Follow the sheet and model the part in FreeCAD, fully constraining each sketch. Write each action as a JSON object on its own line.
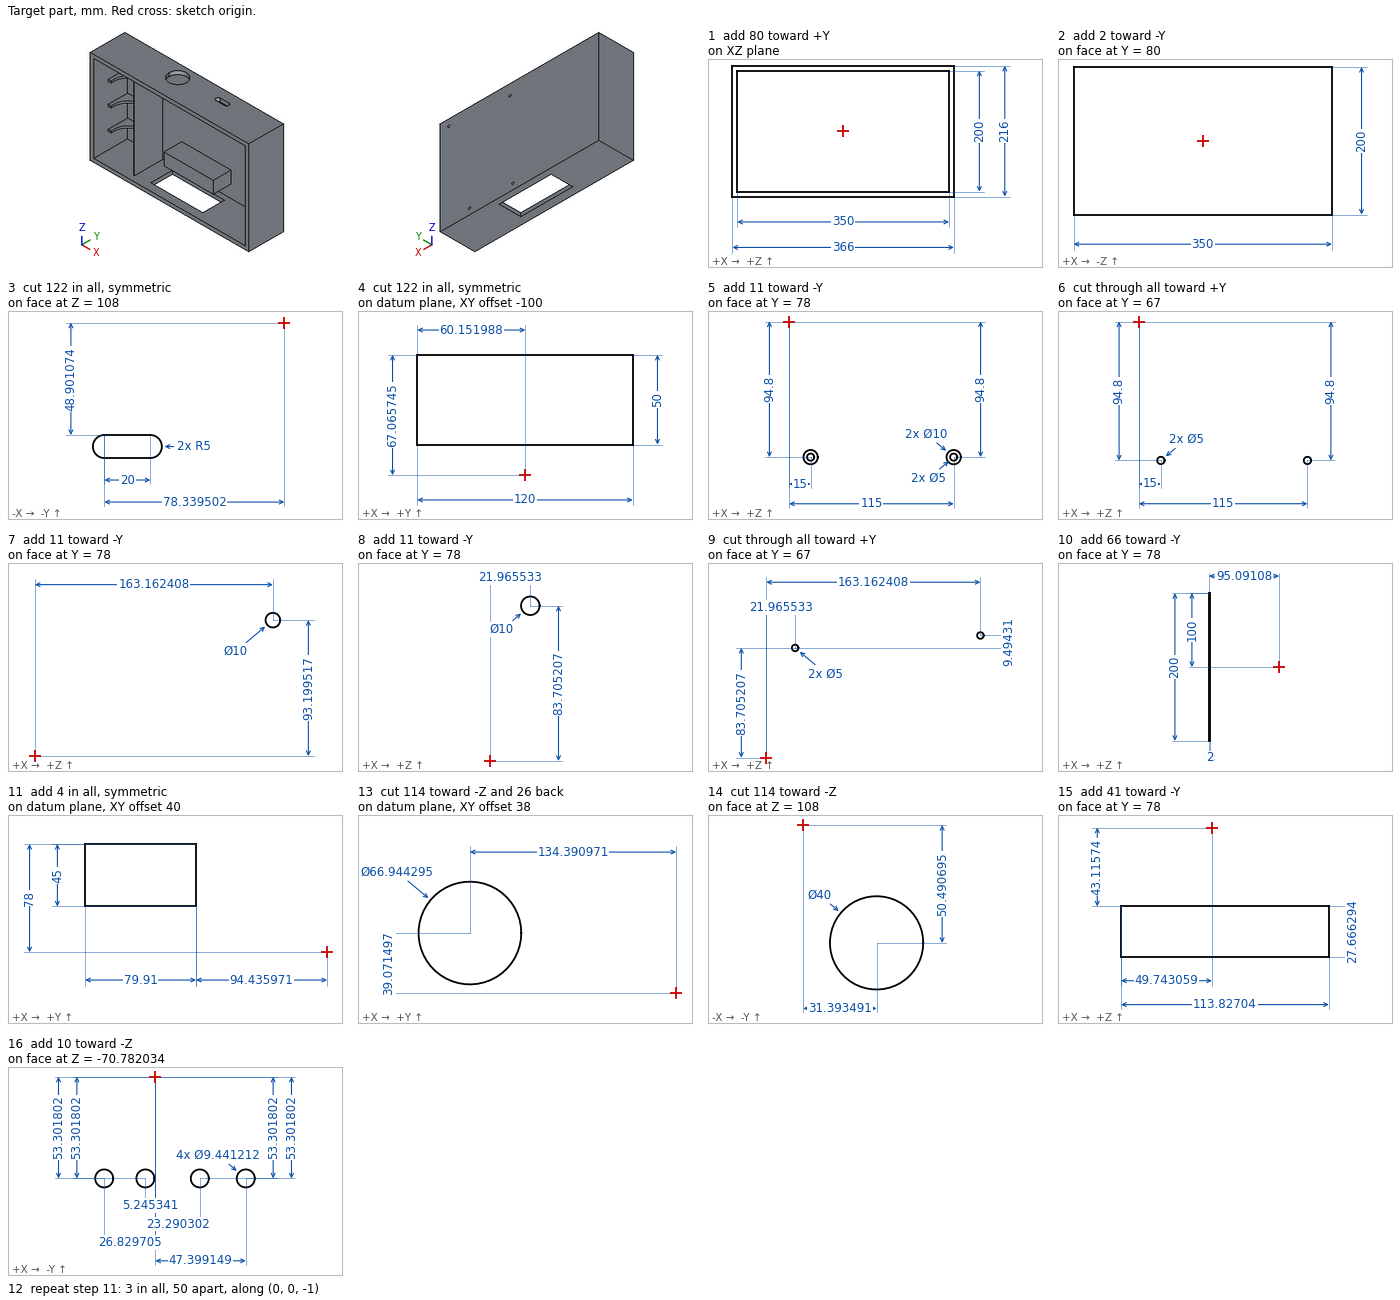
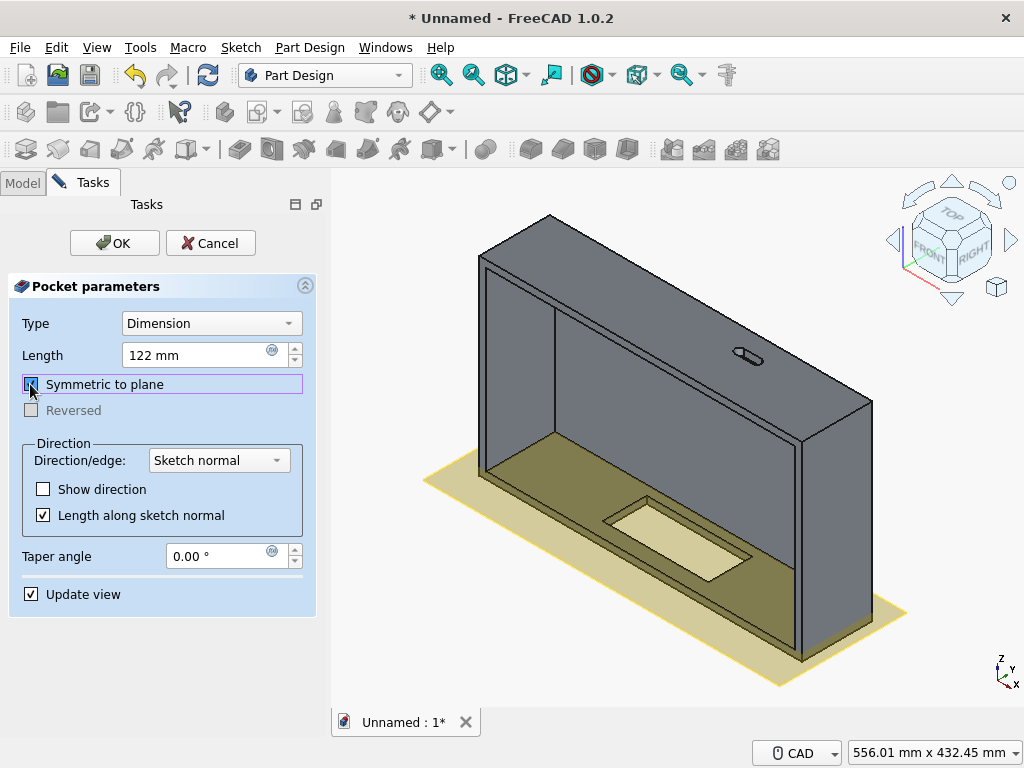
{"action": "left_click", "coordinate": [115, 243]}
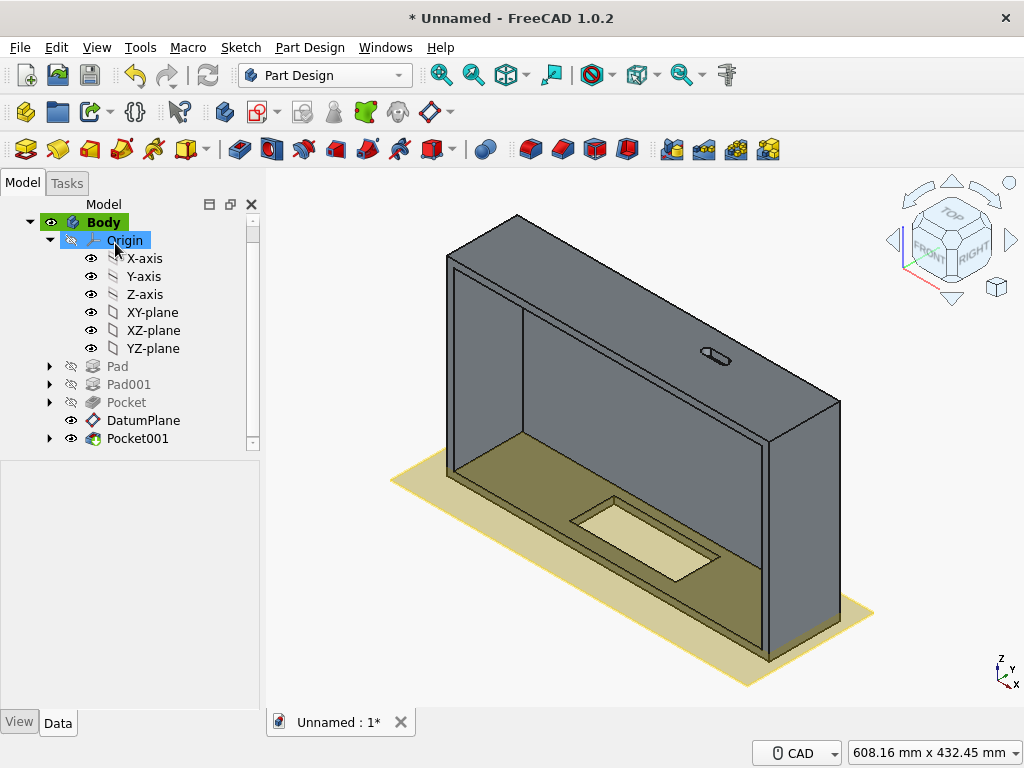
{"action": "left_click", "coordinate": [116, 420]}
{"action": "key", "text": "space"}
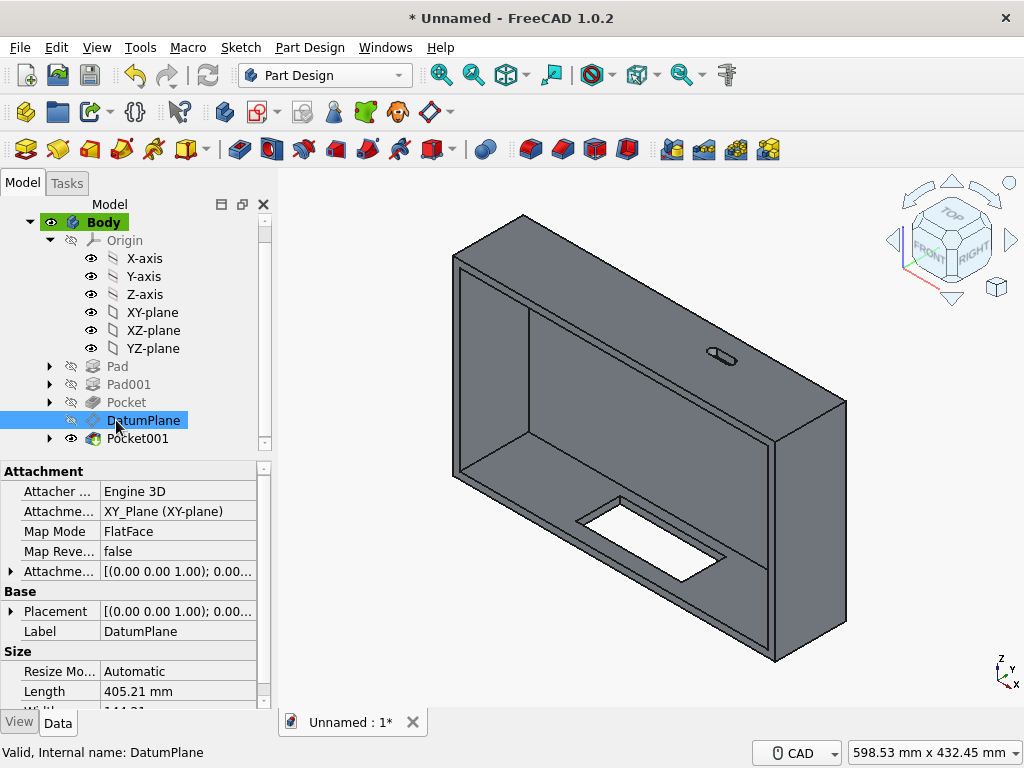
{"action": "left_click", "coordinate": [727, 444]}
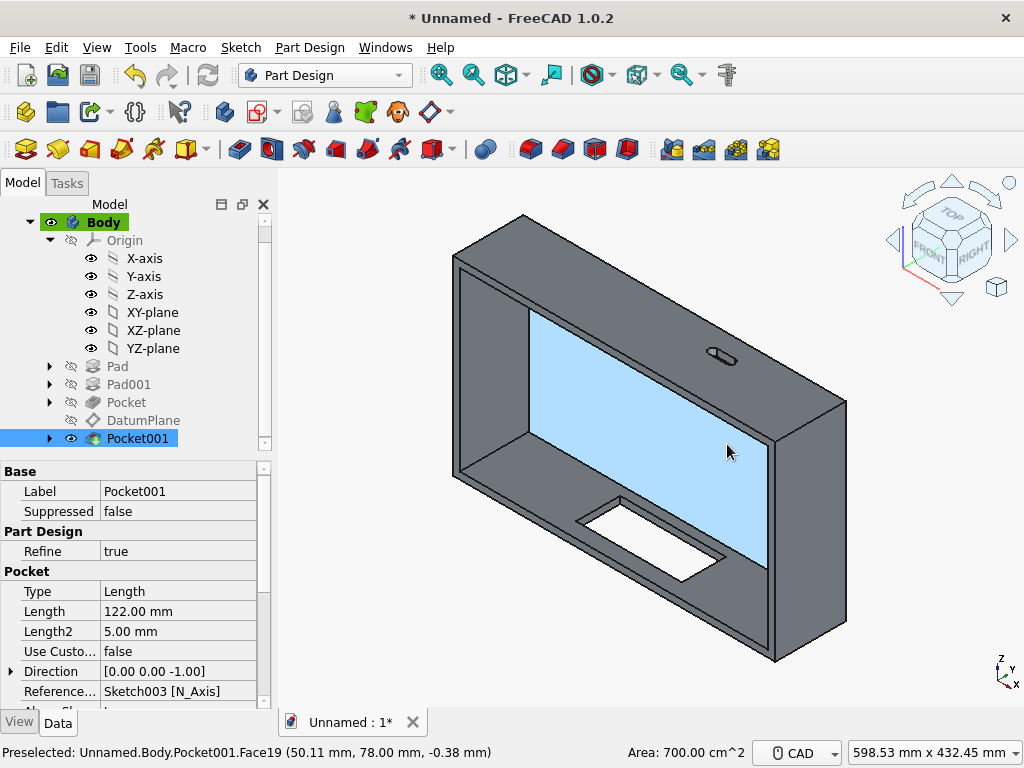
{"action": "left_click", "coordinate": [258, 112]}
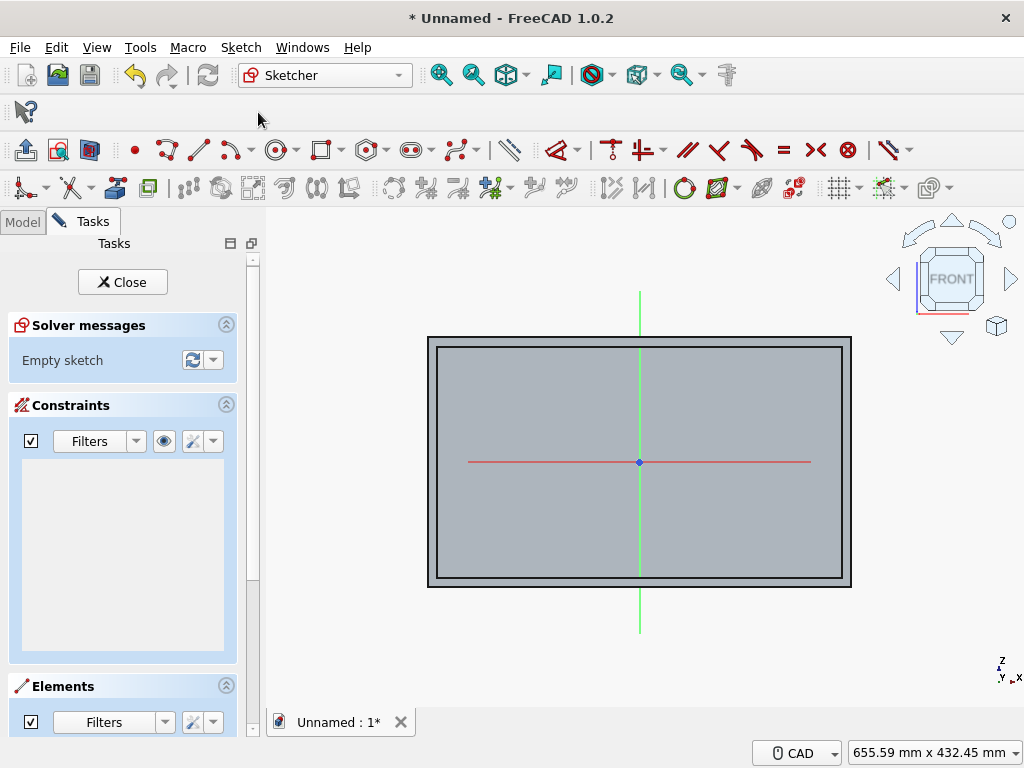
{"action": "left_click", "coordinate": [90, 150]}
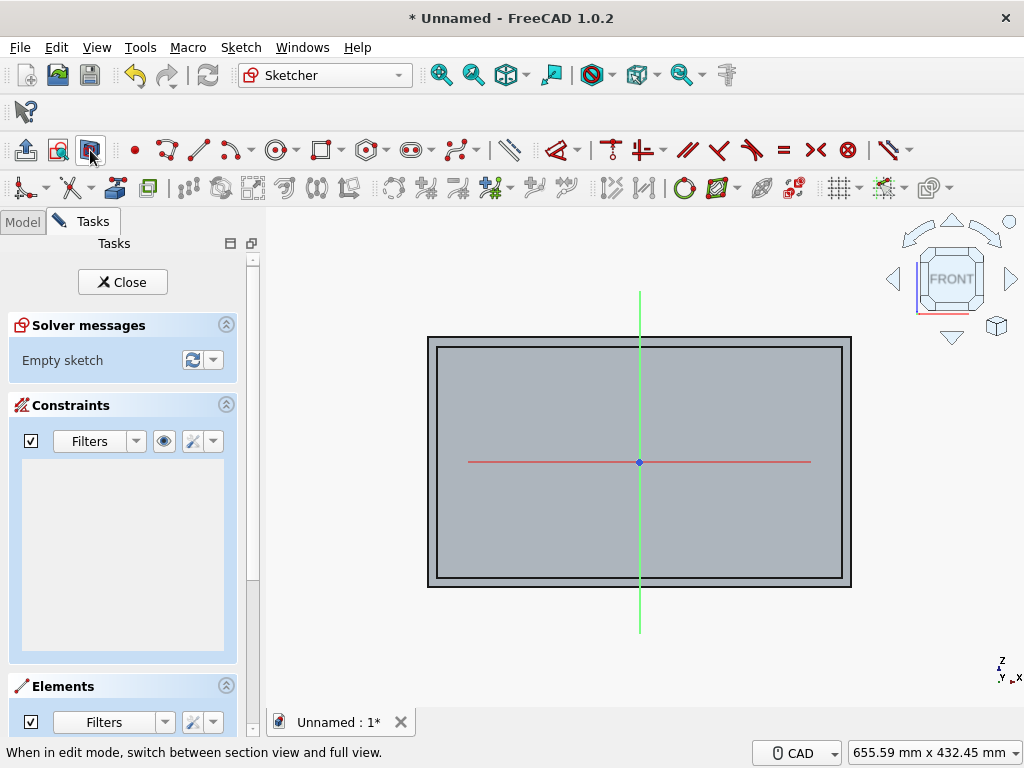
{"action": "scroll", "coordinate": [786, 557], "scroll_direction": "up", "scroll_amount": 5}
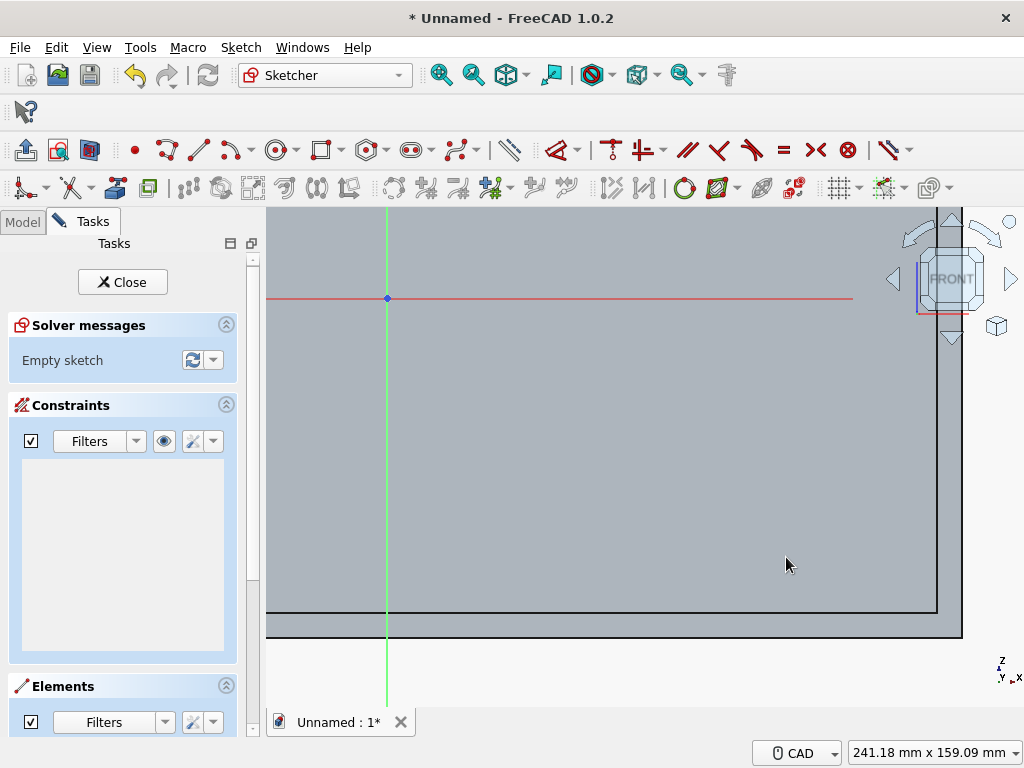
{"action": "key", "text": "g c"}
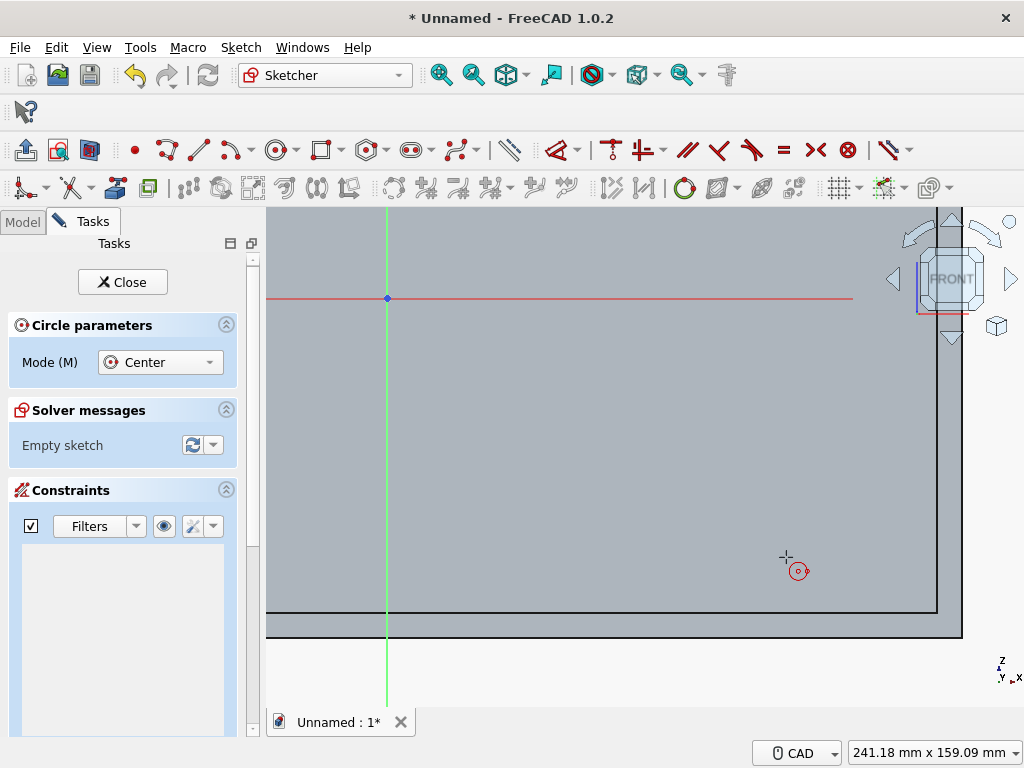
{"action": "scroll", "coordinate": [748, 596], "scroll_direction": "up", "scroll_amount": 2}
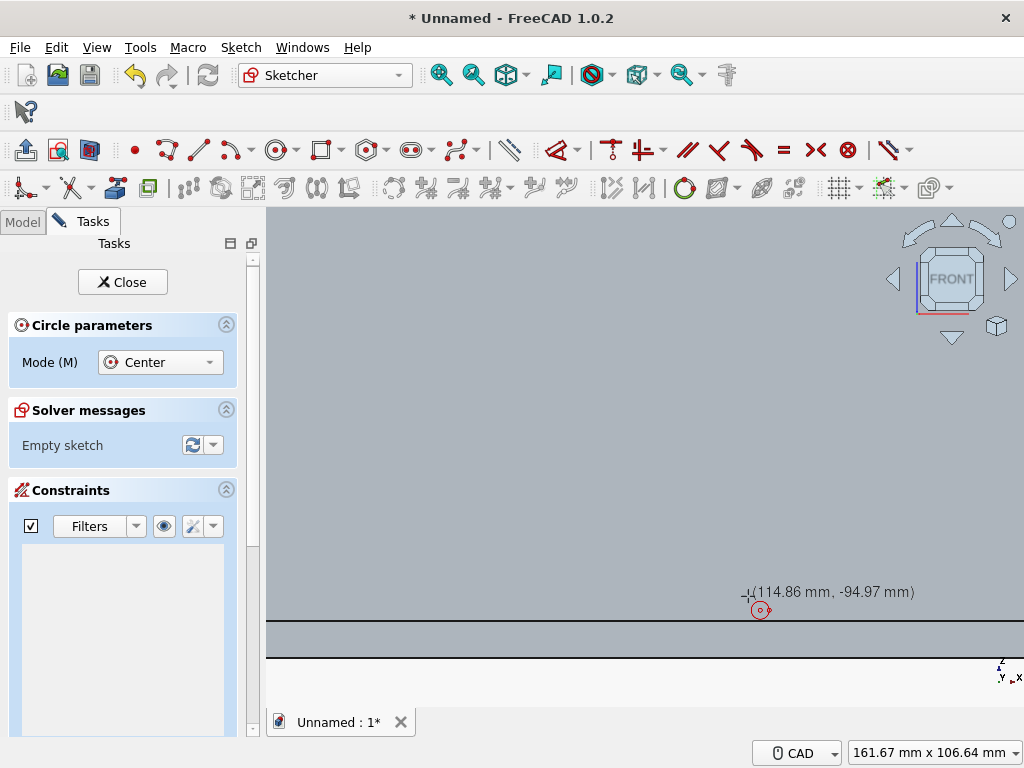
{"action": "left_click", "coordinate": [748, 596]}
{"action": "mouse_move", "coordinate": [765, 580]}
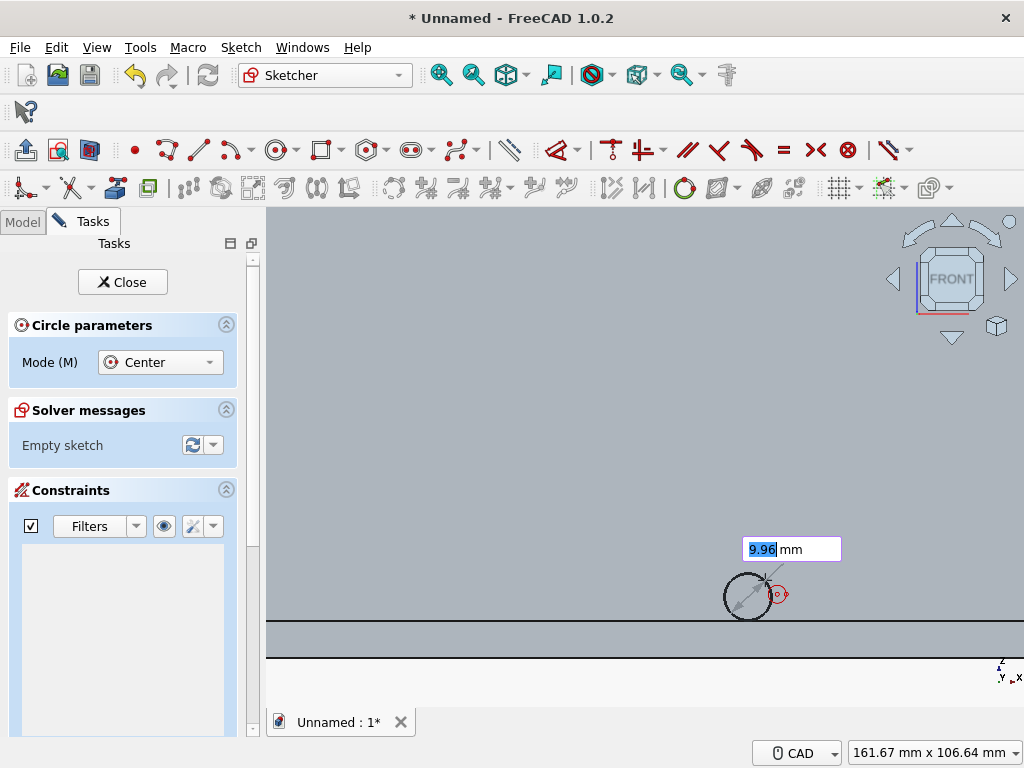
{"action": "type", "text": "10"}
{"action": "key", "text": "Return"}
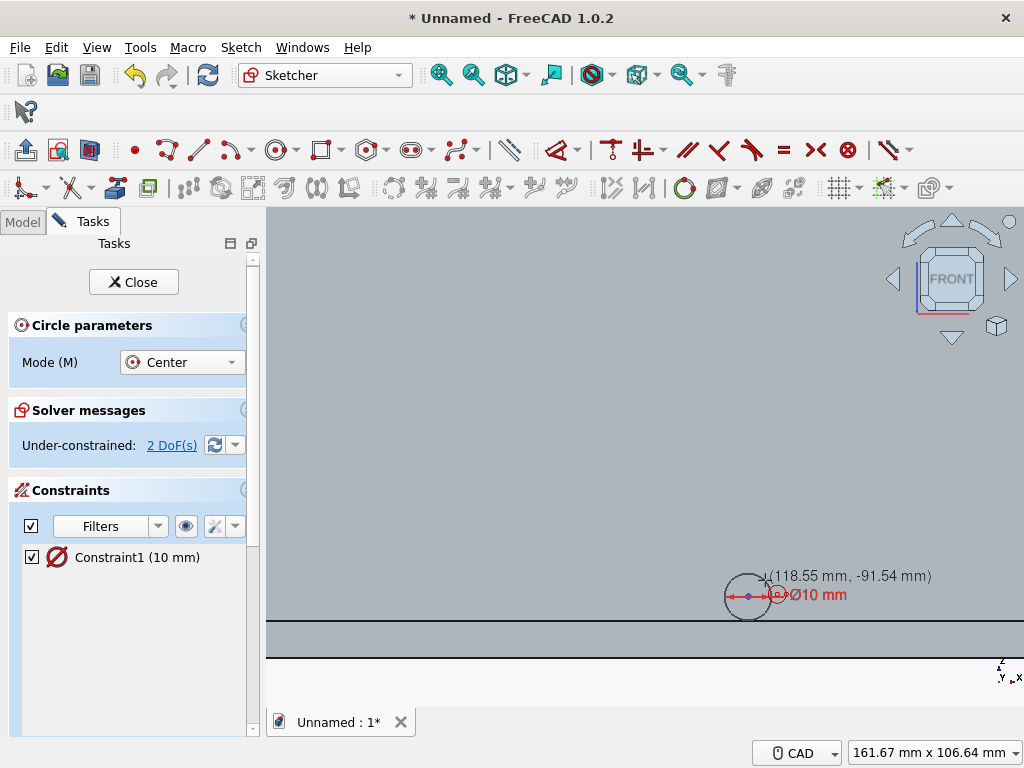
{"action": "scroll", "coordinate": [751, 602], "scroll_direction": "down", "scroll_amount": 2}